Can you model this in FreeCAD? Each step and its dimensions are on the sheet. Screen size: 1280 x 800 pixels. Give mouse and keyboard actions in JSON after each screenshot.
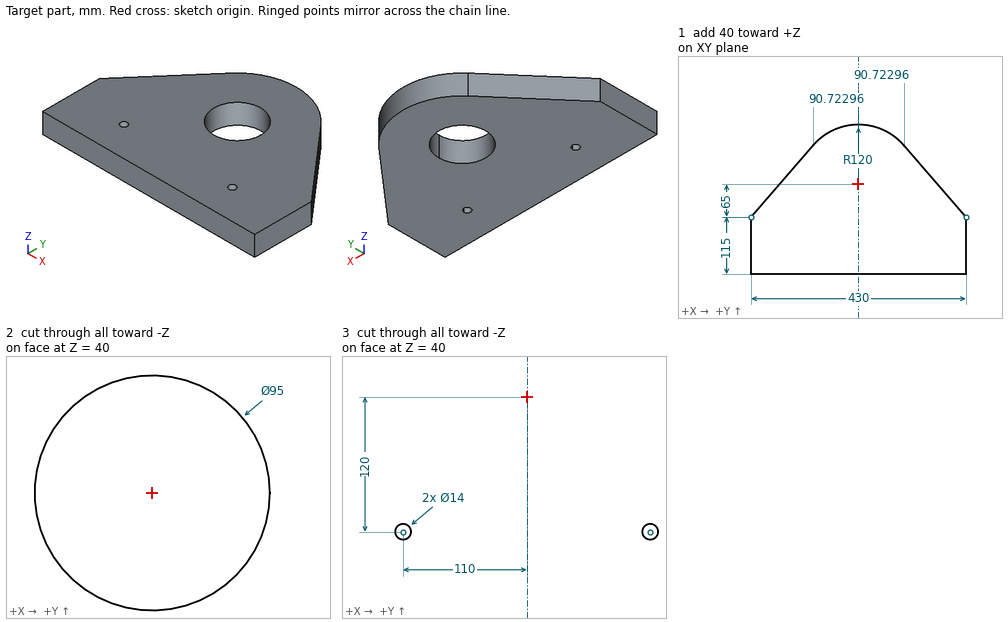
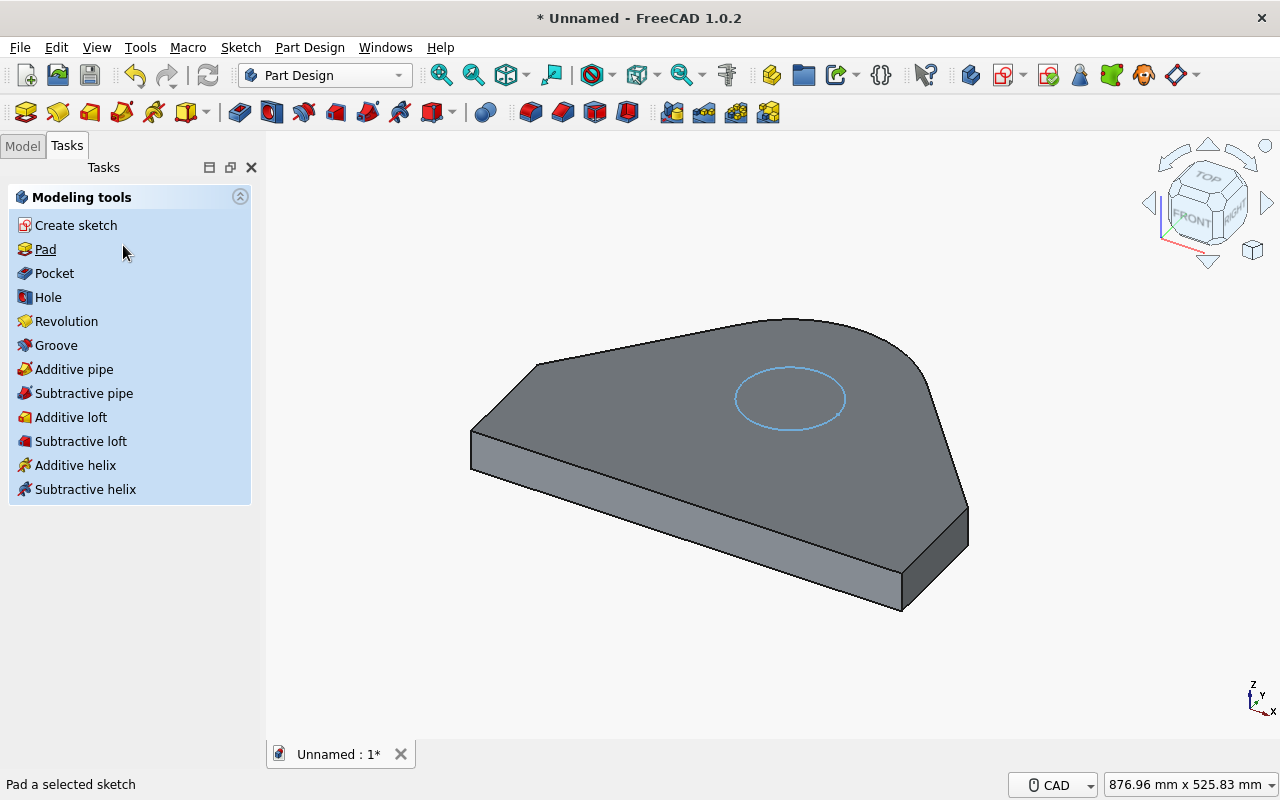
{"action": "left_click", "coordinate": [240, 112]}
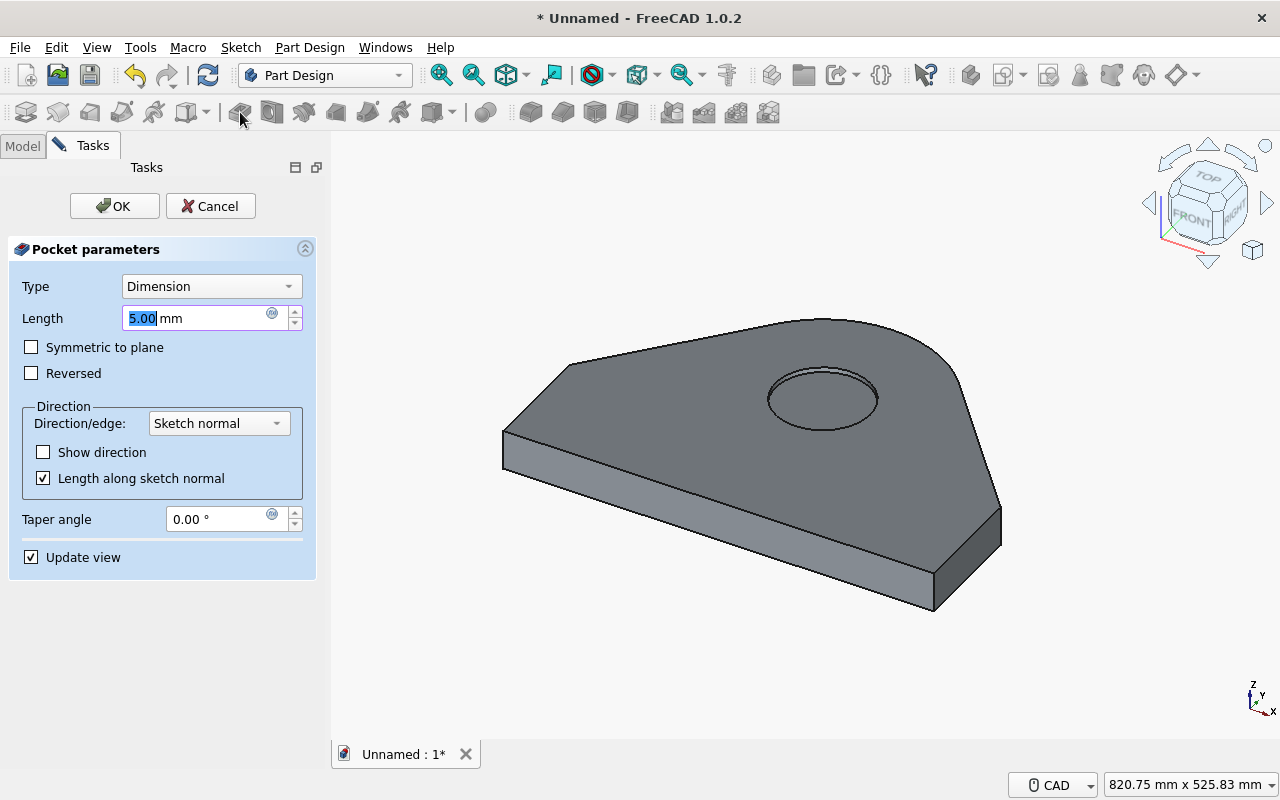
{"action": "left_click", "coordinate": [212, 286]}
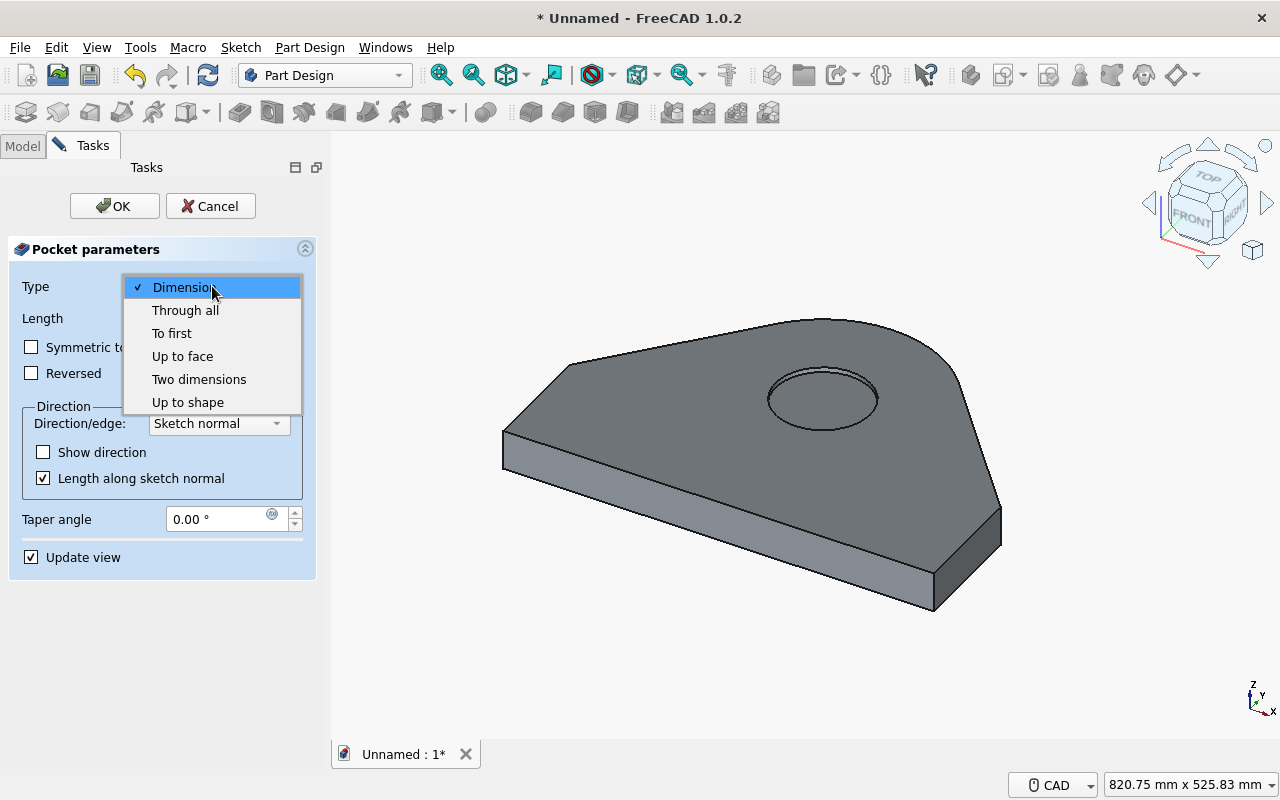
{"action": "left_click", "coordinate": [212, 310]}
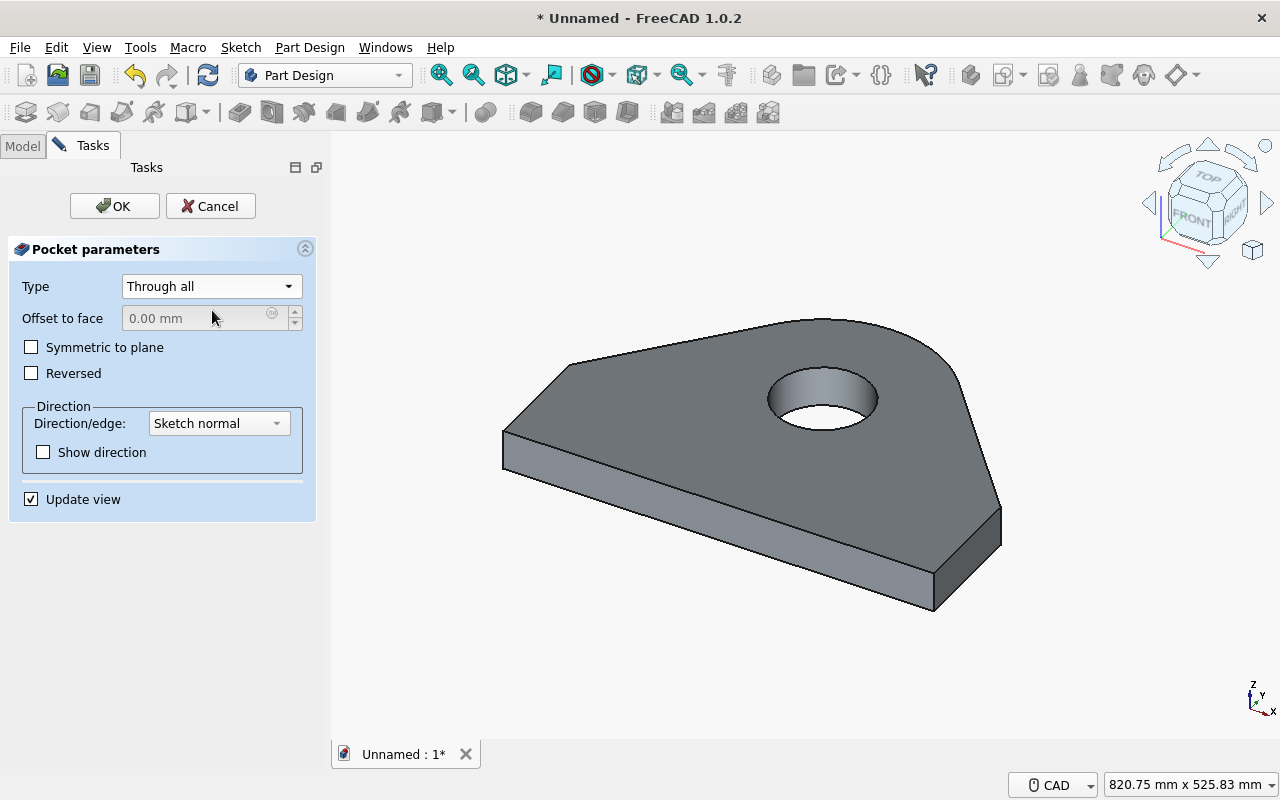
{"action": "left_click", "coordinate": [115, 206]}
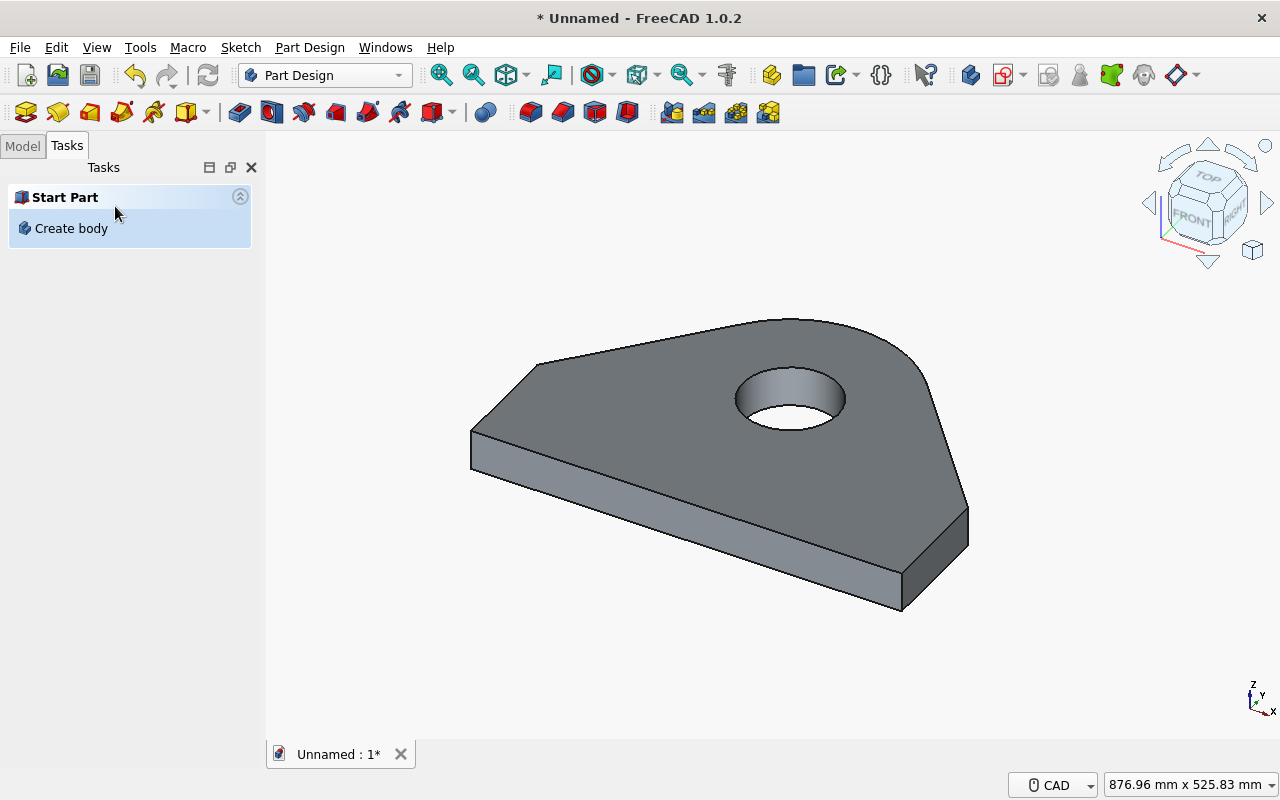
{"action": "left_click", "coordinate": [871, 480]}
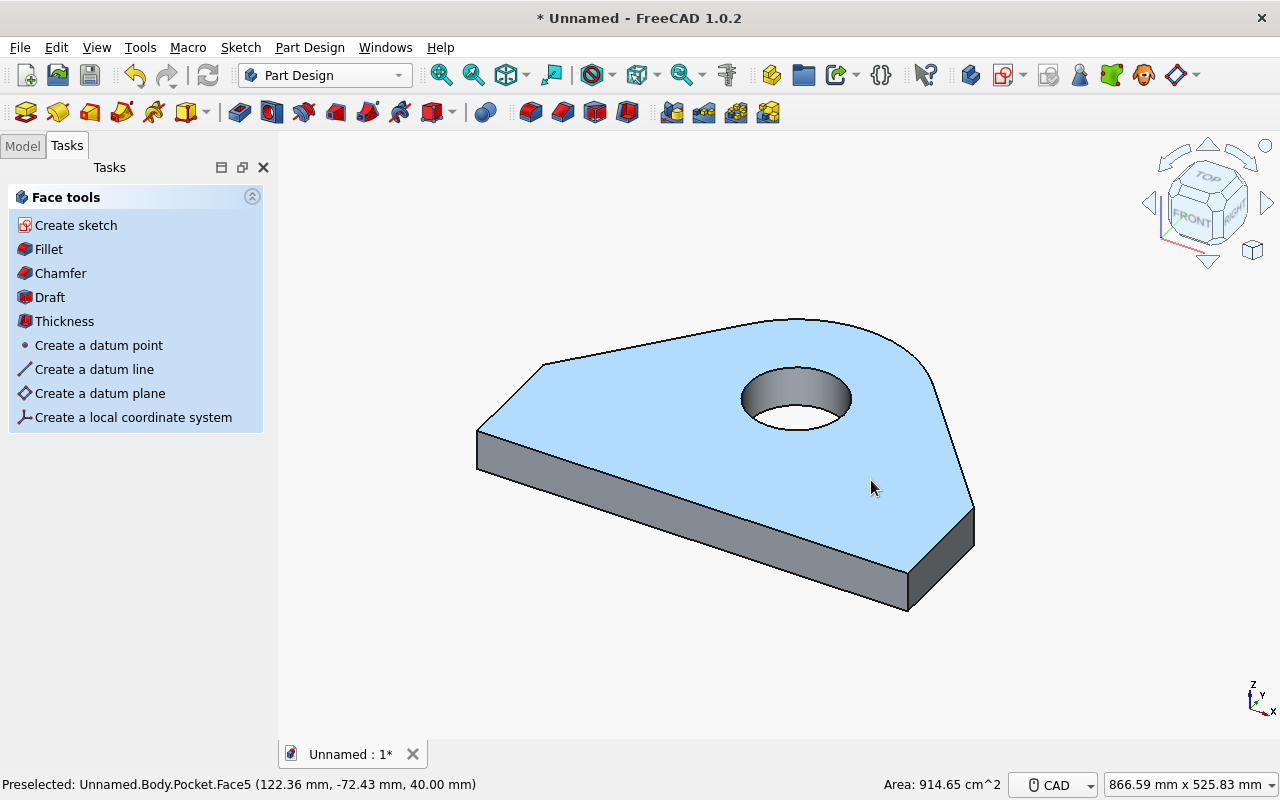
{"action": "left_click", "coordinate": [1004, 76]}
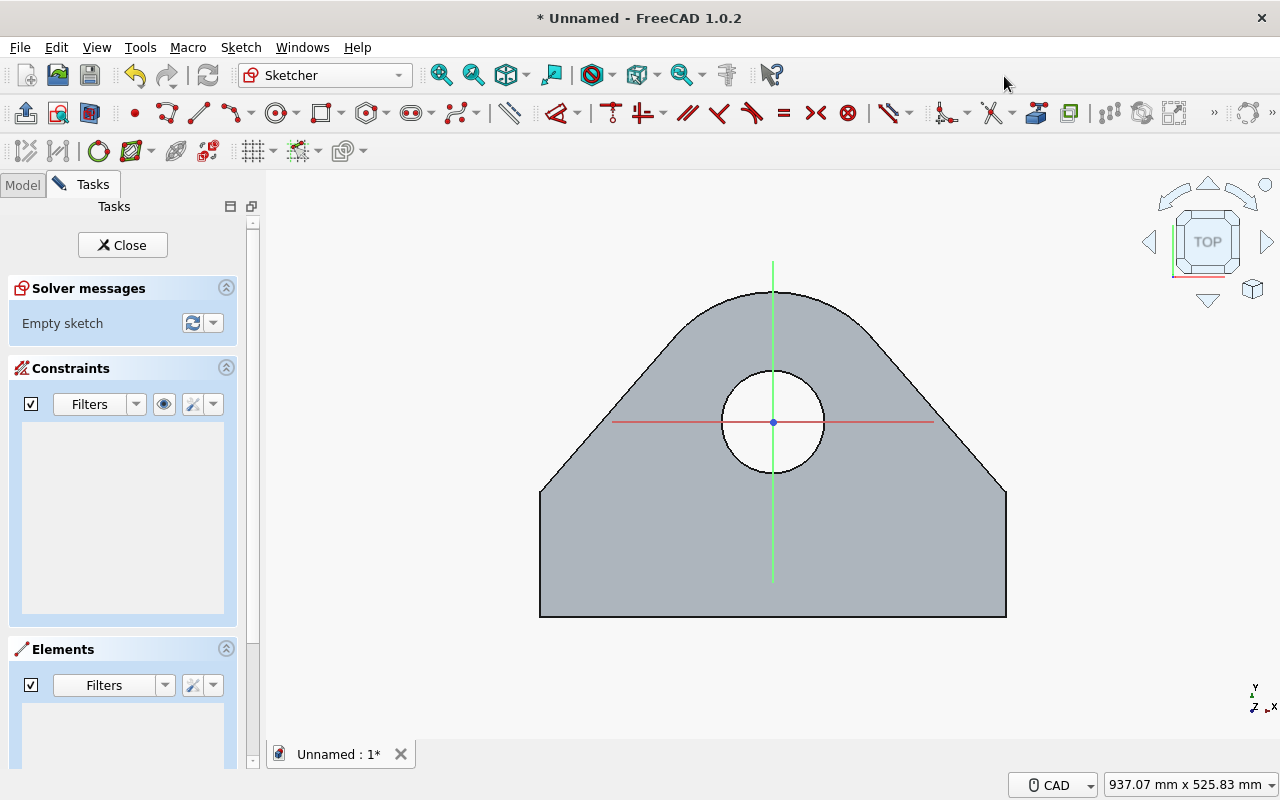
{"action": "scroll", "coordinate": [829, 520], "scroll_direction": "up", "scroll_amount": 4}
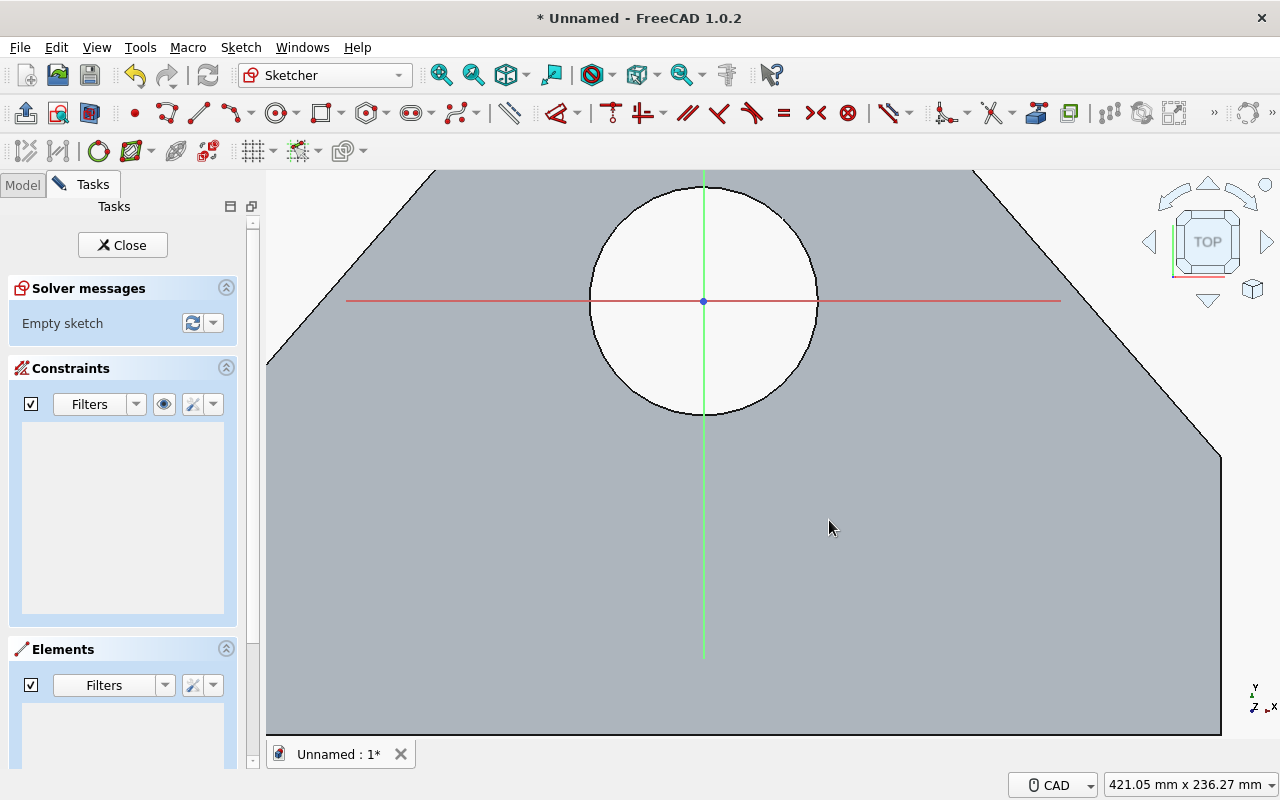
{"action": "left_click", "coordinate": [276, 114]}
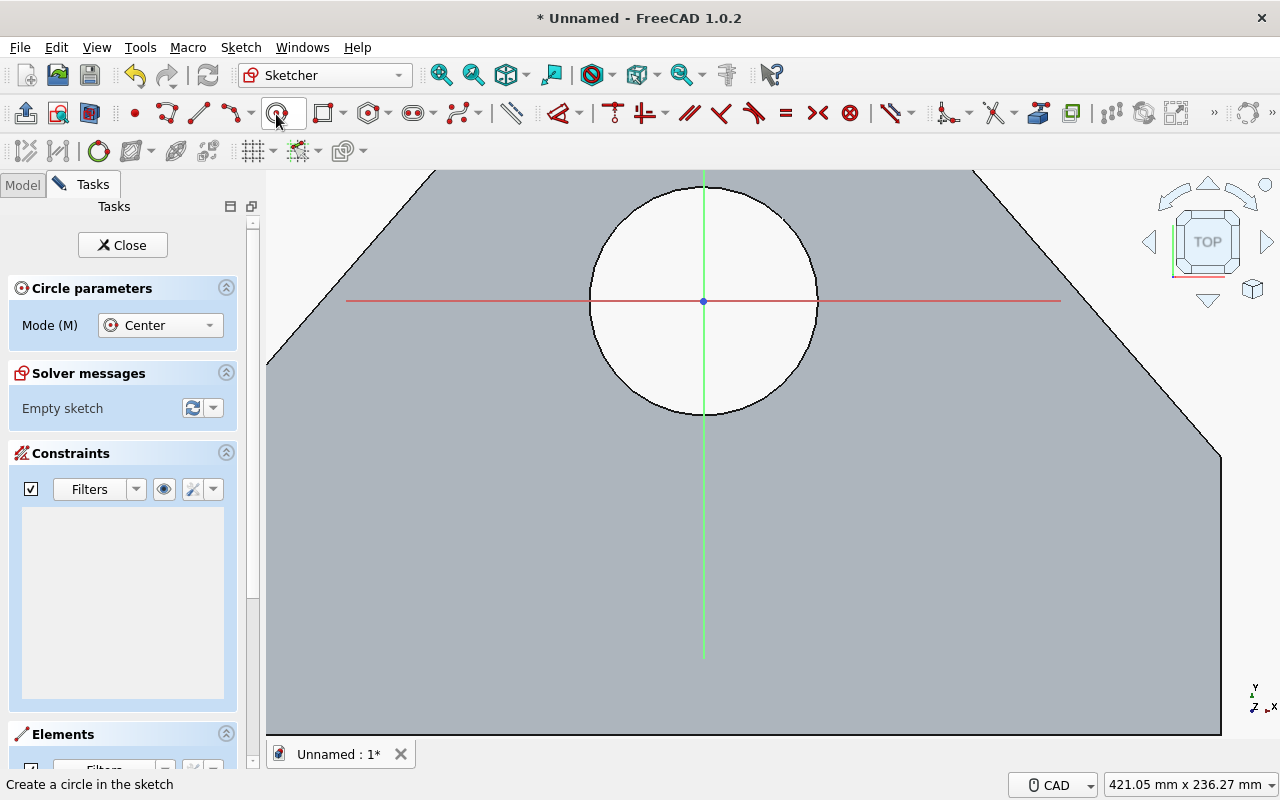
{"action": "scroll", "coordinate": [439, 590], "scroll_direction": "up", "scroll_amount": 2}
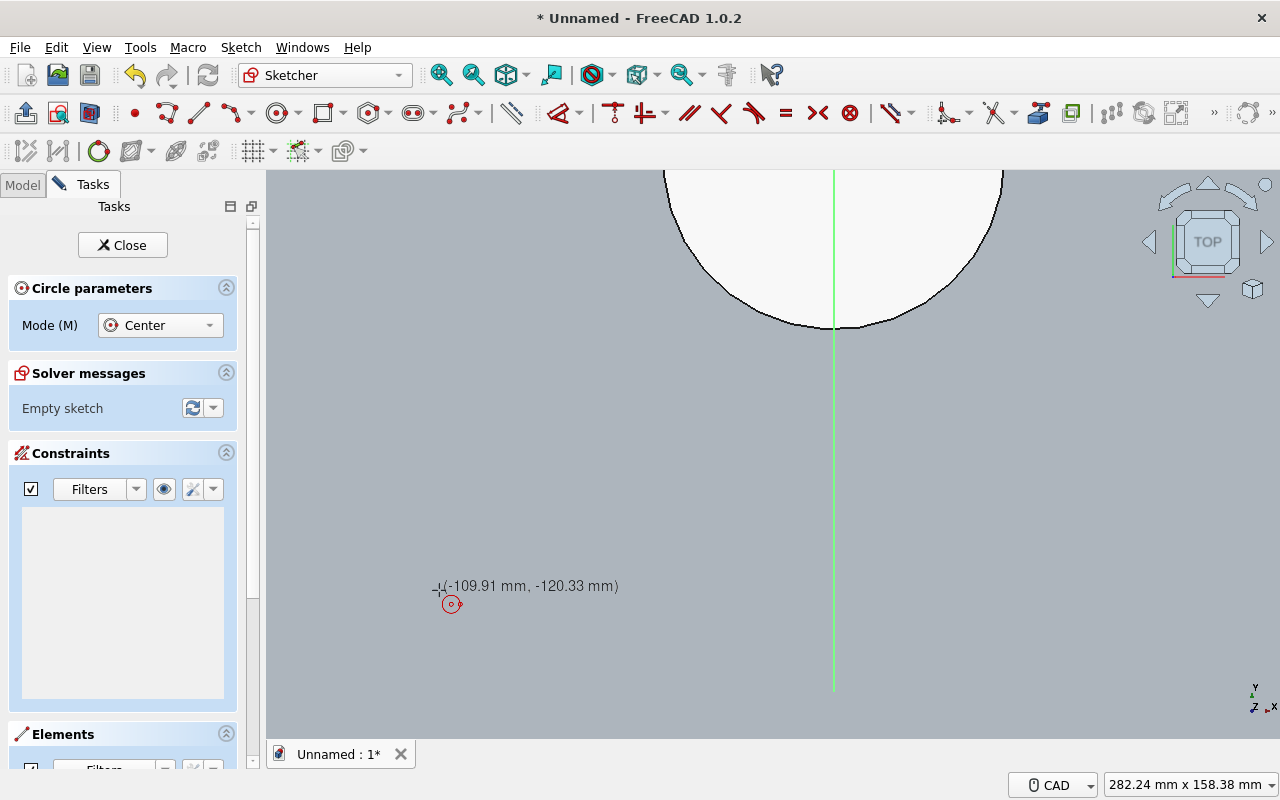
{"action": "left_click", "coordinate": [439, 590]}
{"action": "mouse_move", "coordinate": [456, 572]}